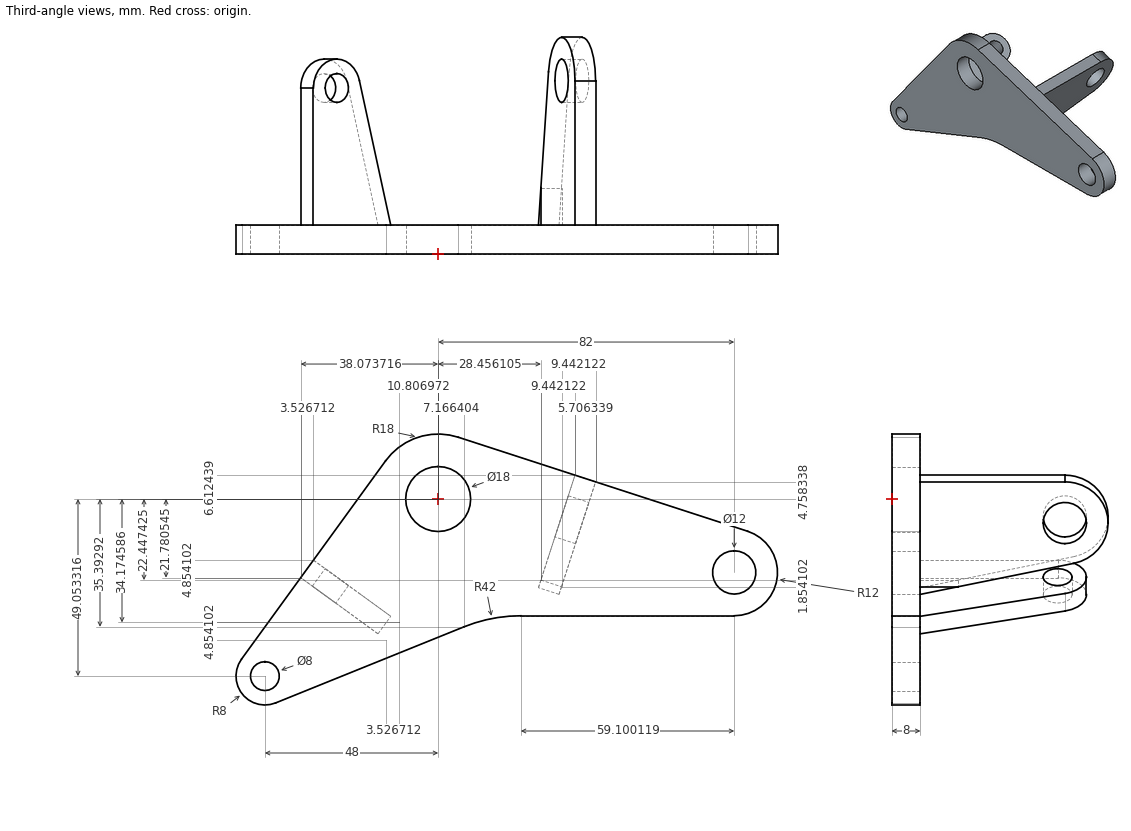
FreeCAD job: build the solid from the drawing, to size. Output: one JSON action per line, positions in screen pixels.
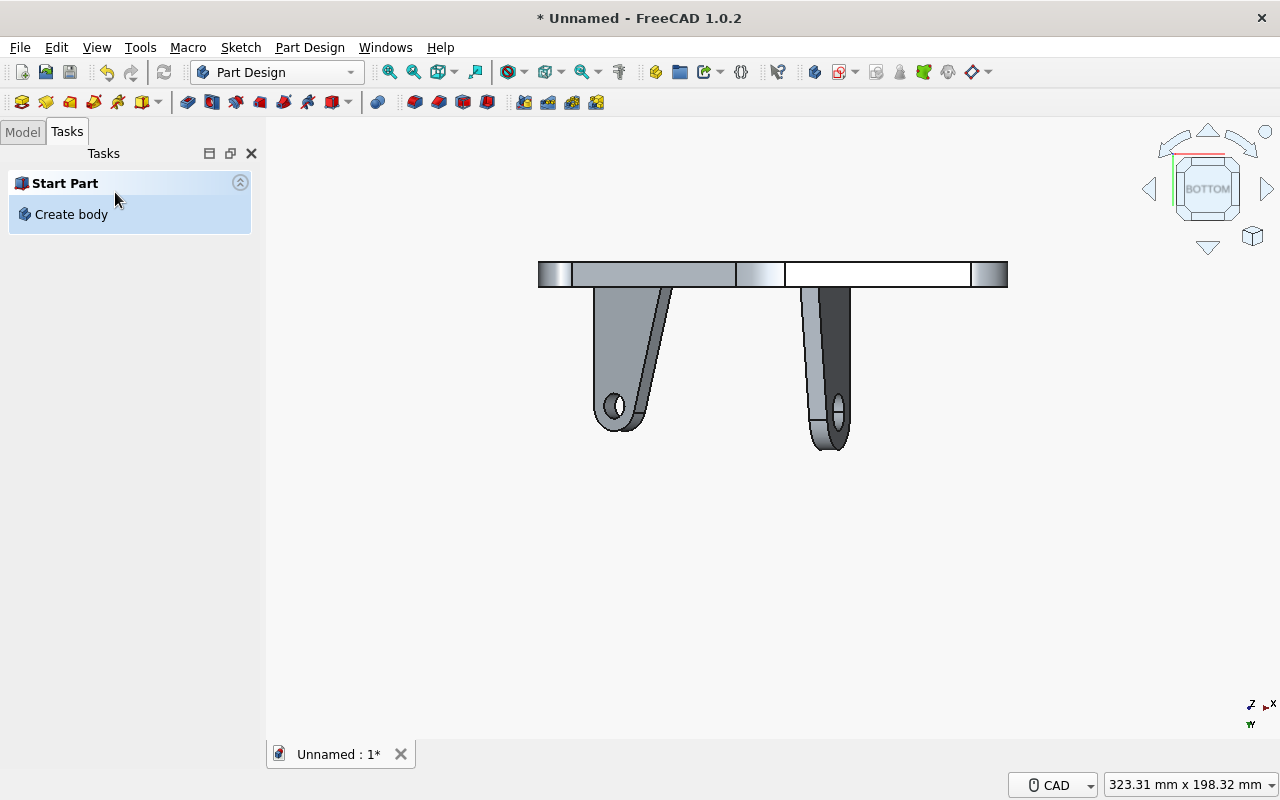
{"action": "key", "text": "0"}